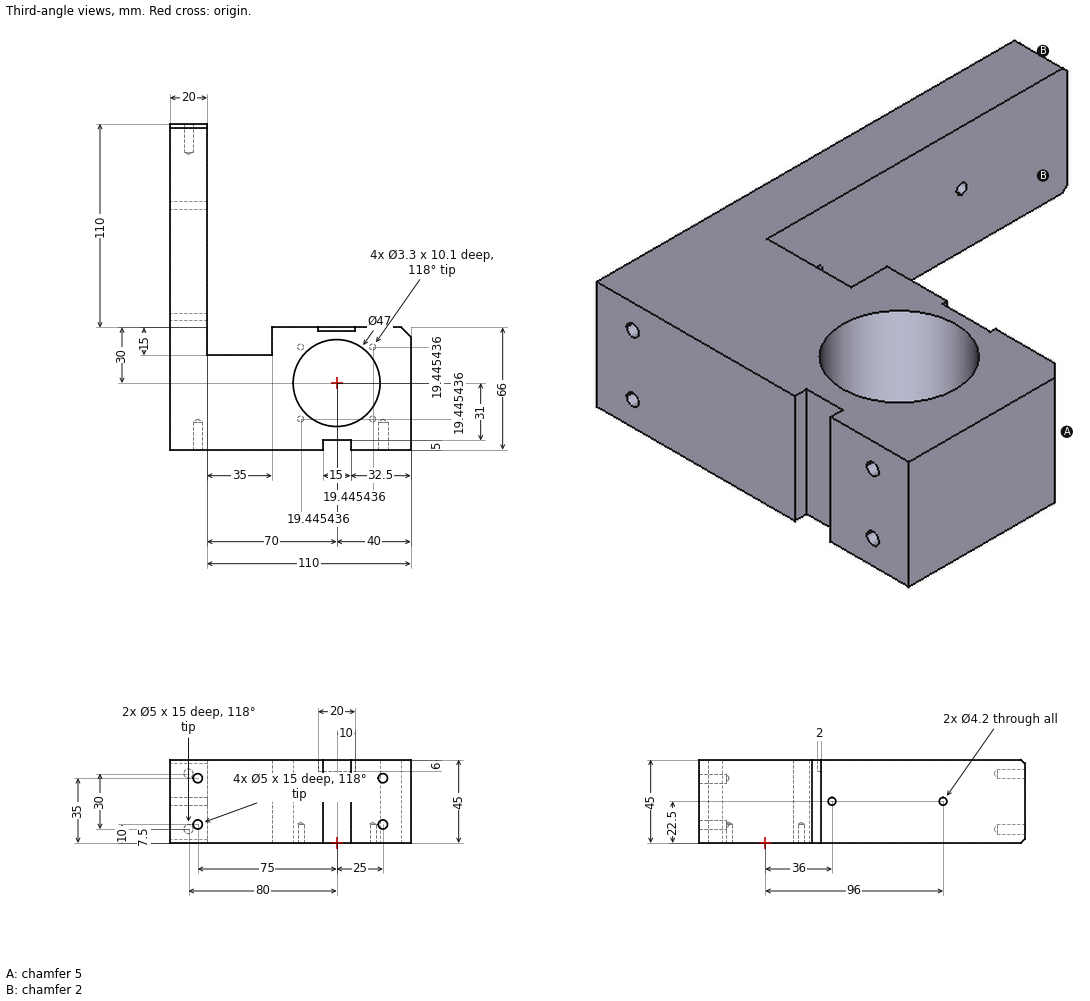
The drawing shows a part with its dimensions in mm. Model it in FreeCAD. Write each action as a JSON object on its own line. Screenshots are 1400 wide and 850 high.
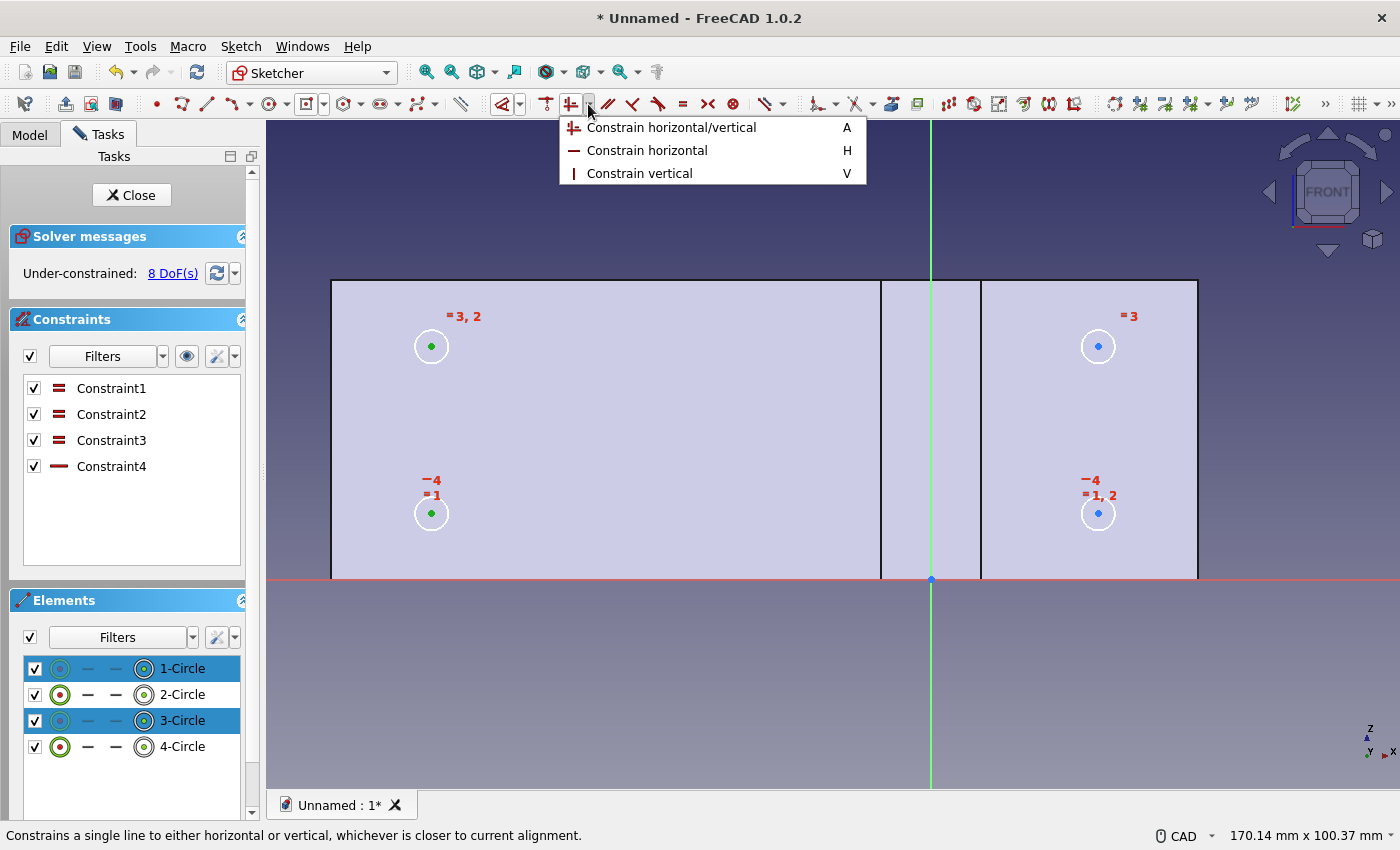
{"action": "left_click", "coordinate": [713, 174]}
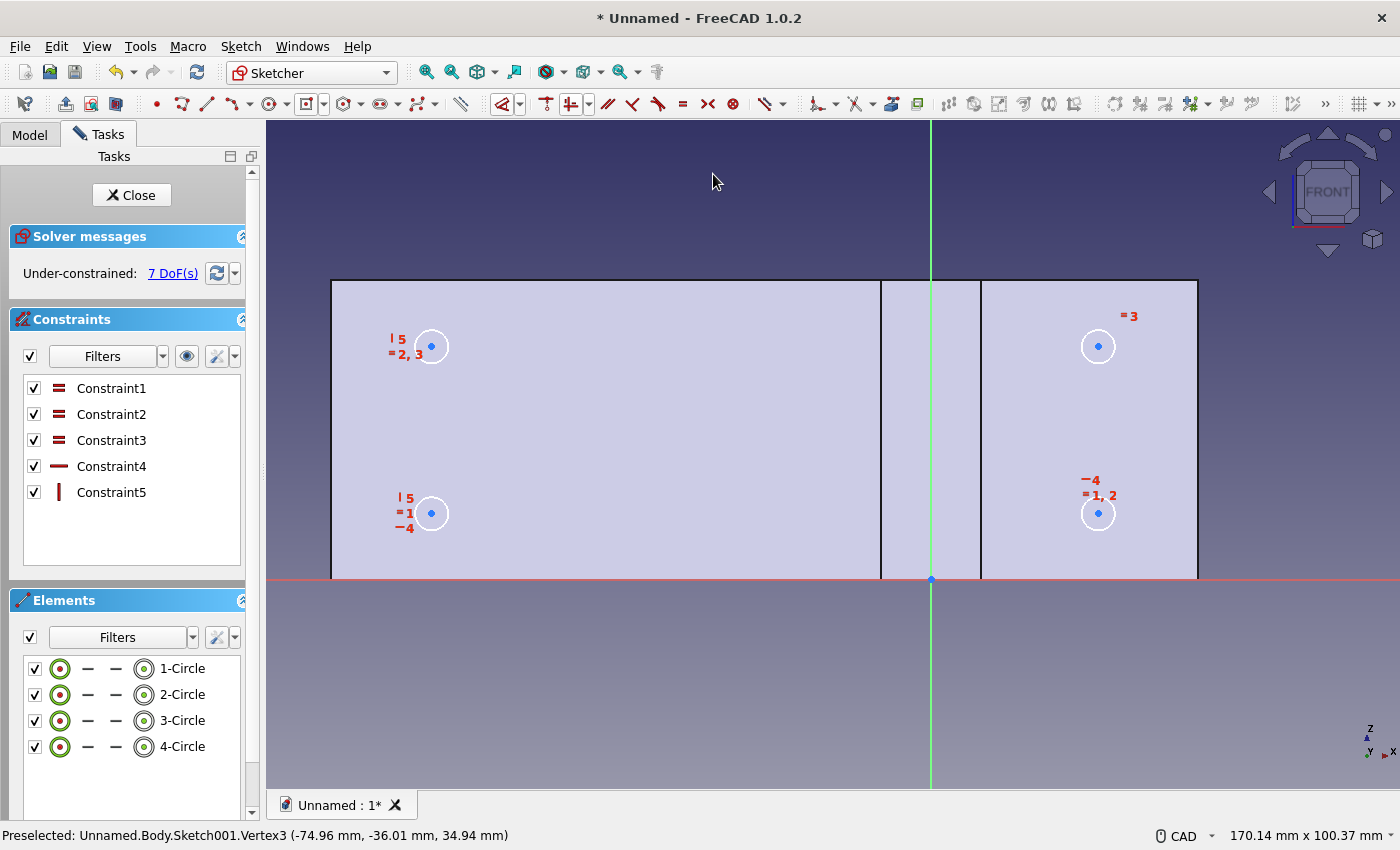
{"action": "left_click", "coordinate": [1098, 514]}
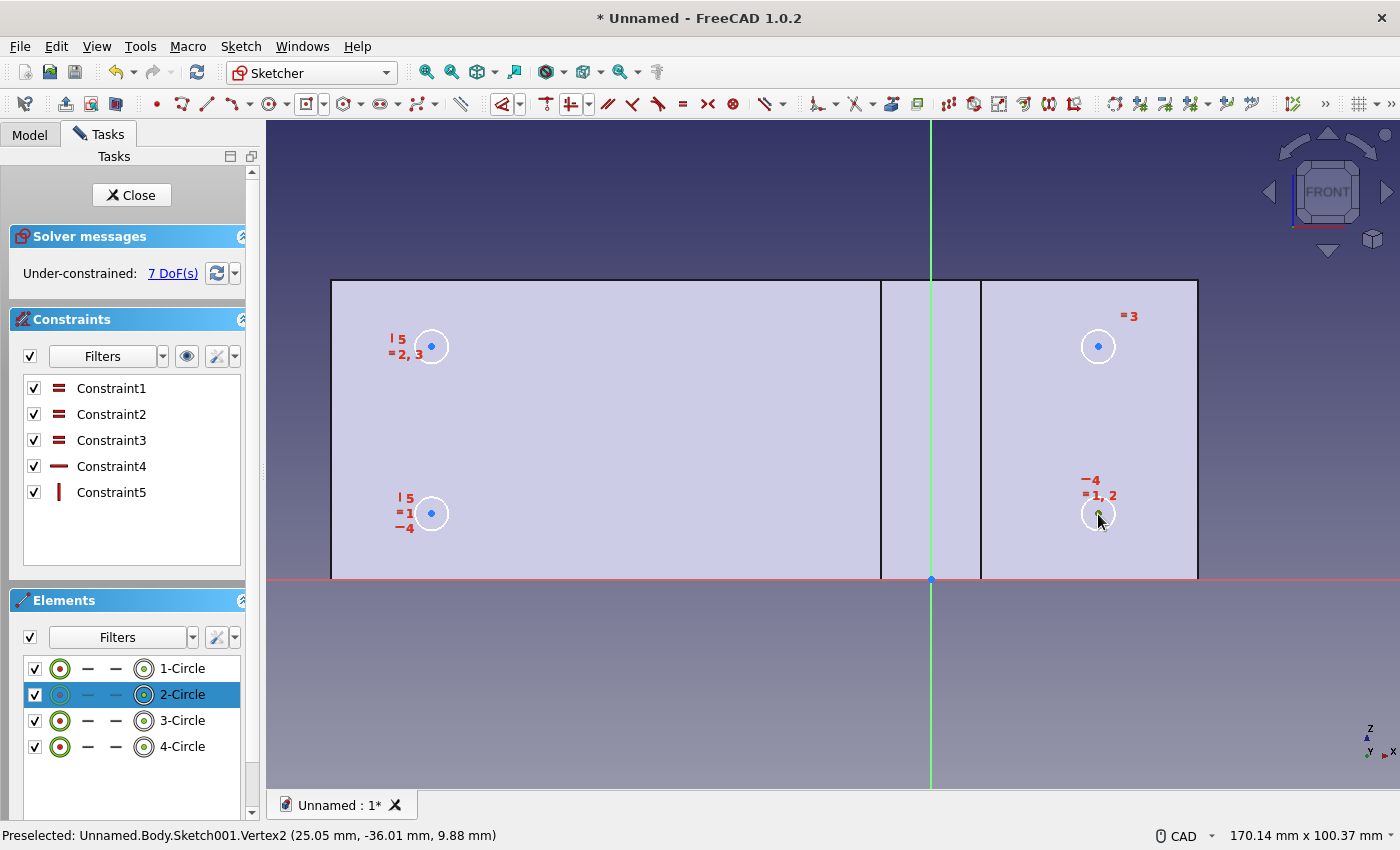
{"action": "left_click", "coordinate": [1098, 347]}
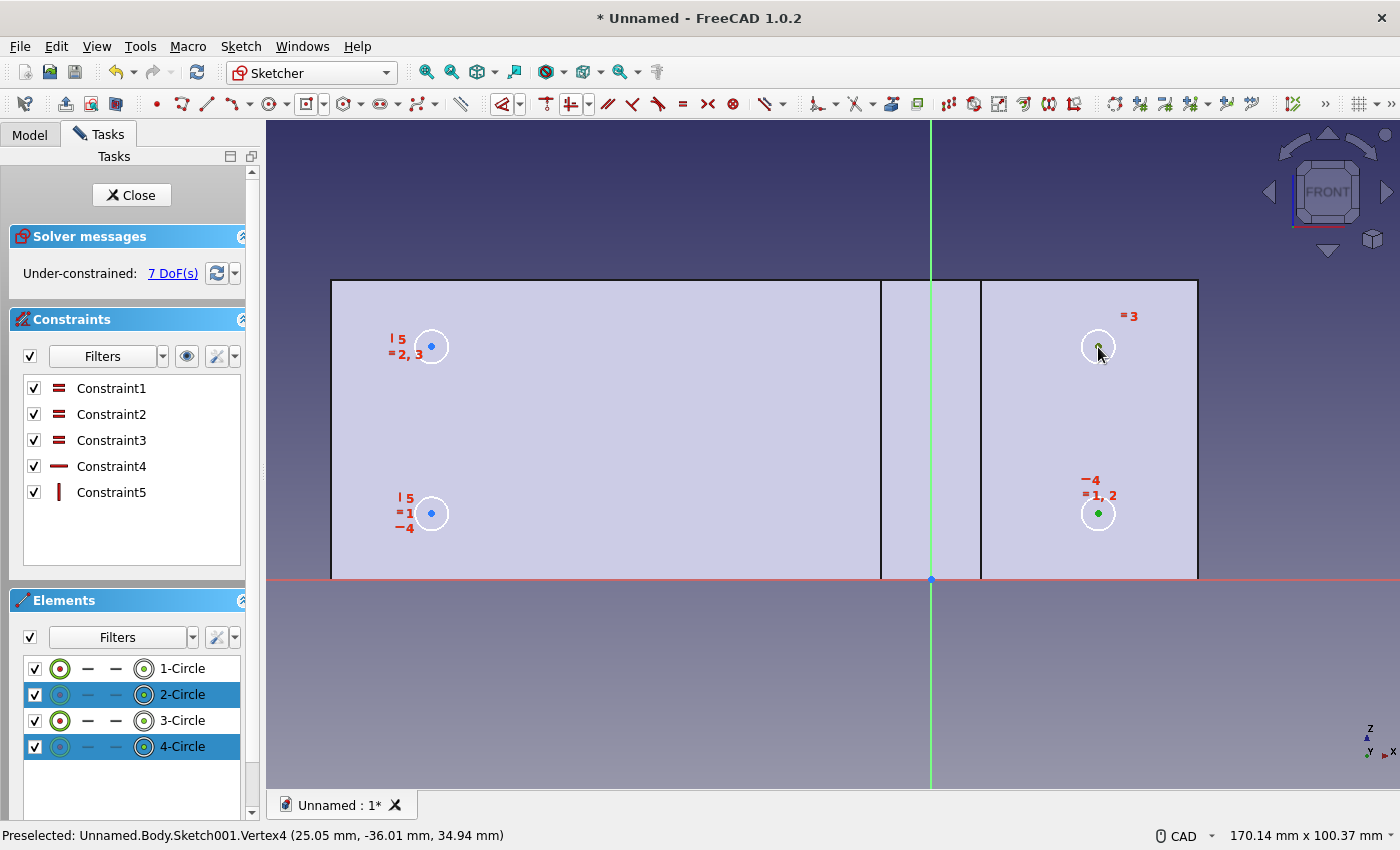
{"action": "left_click", "coordinate": [588, 104]}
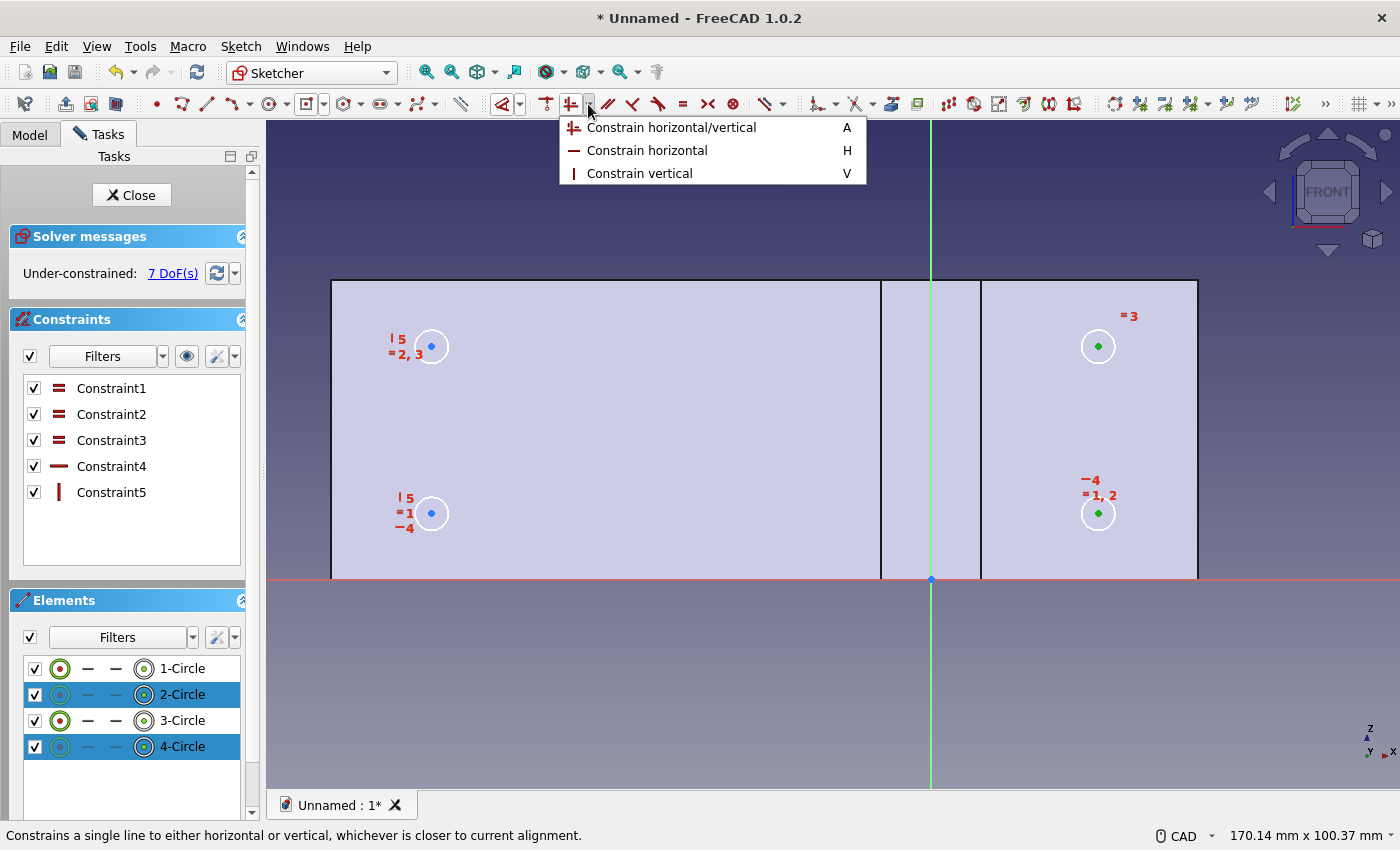
{"action": "left_click", "coordinate": [713, 174]}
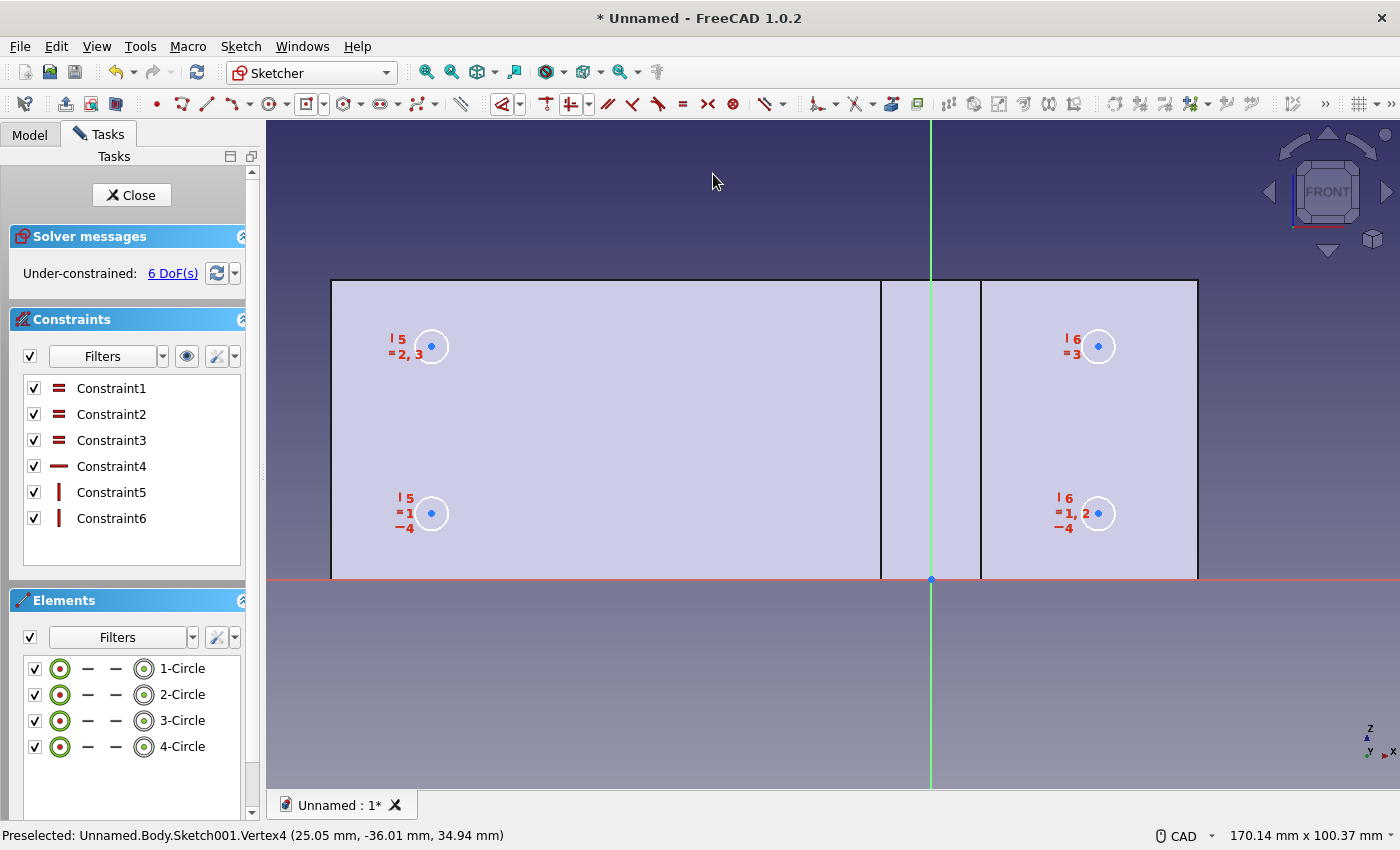
{"action": "left_click", "coordinate": [432, 347]}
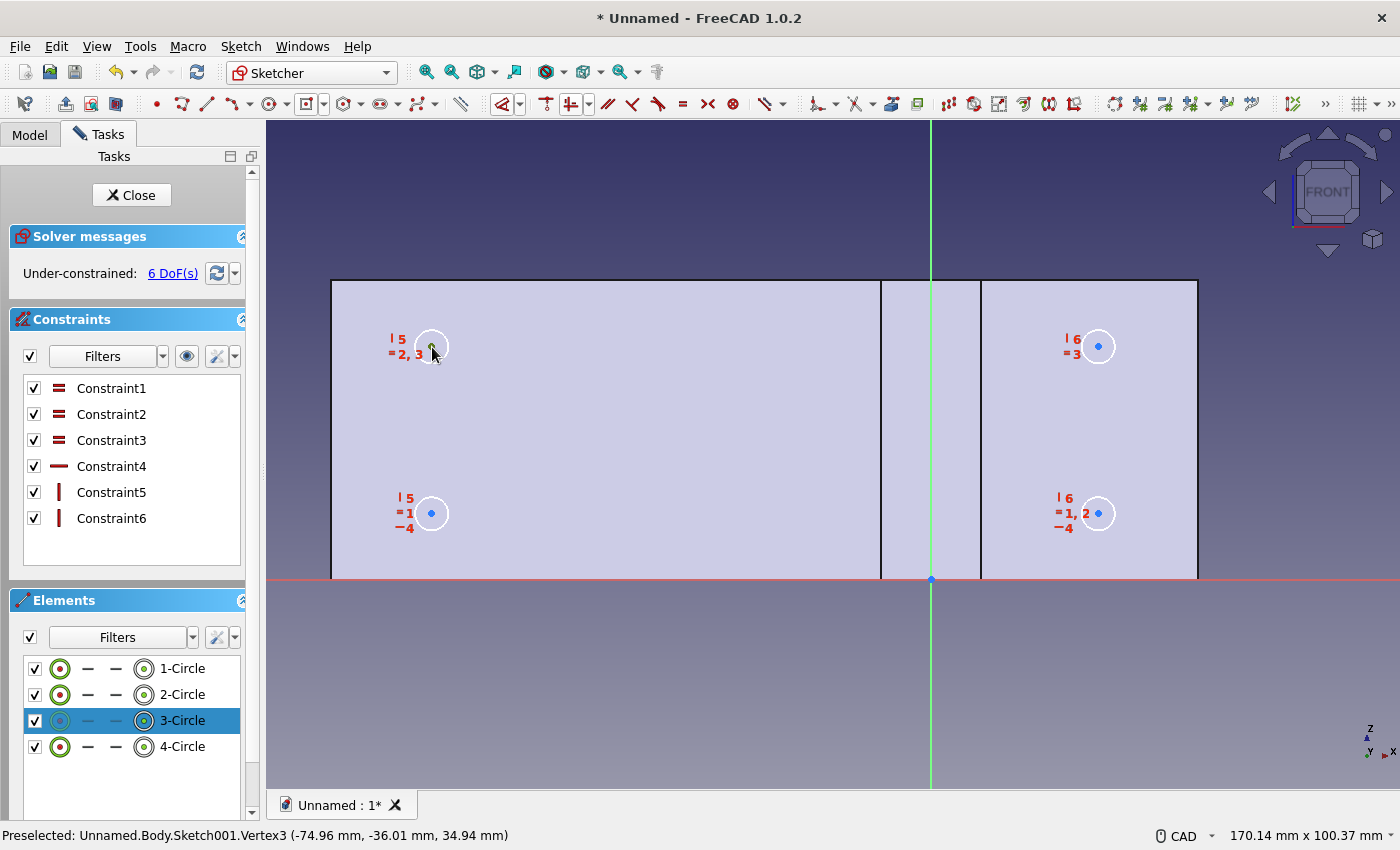
{"action": "left_click", "coordinate": [1098, 347]}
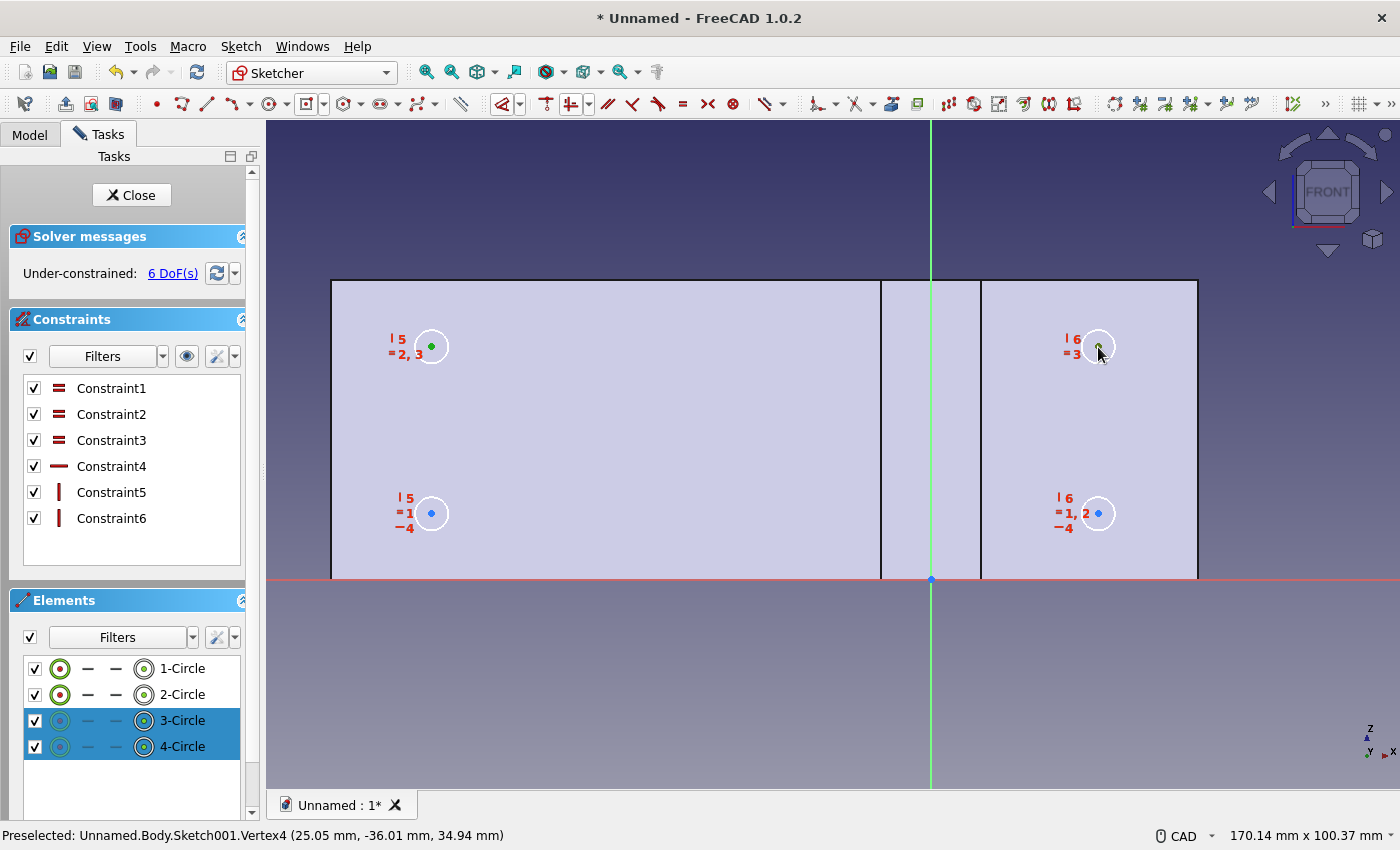
{"action": "key", "text": "h"}